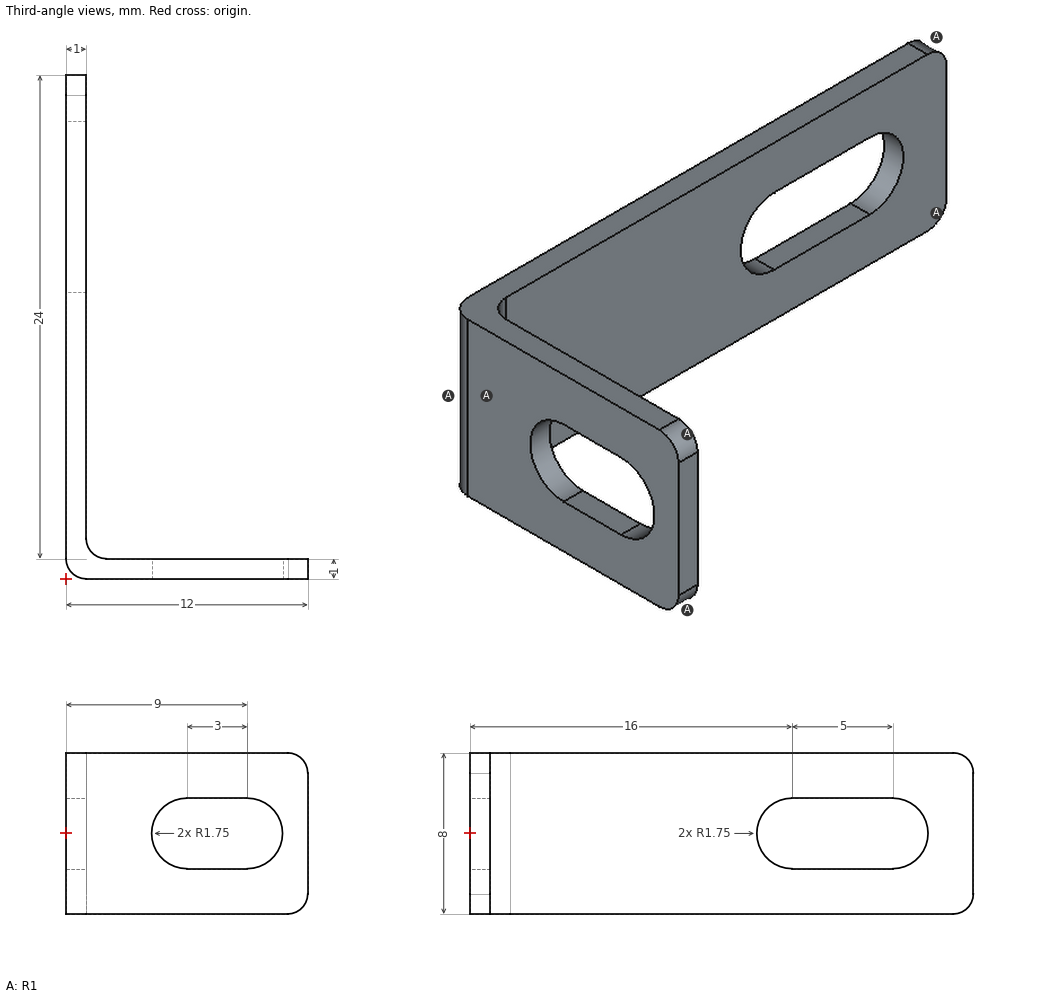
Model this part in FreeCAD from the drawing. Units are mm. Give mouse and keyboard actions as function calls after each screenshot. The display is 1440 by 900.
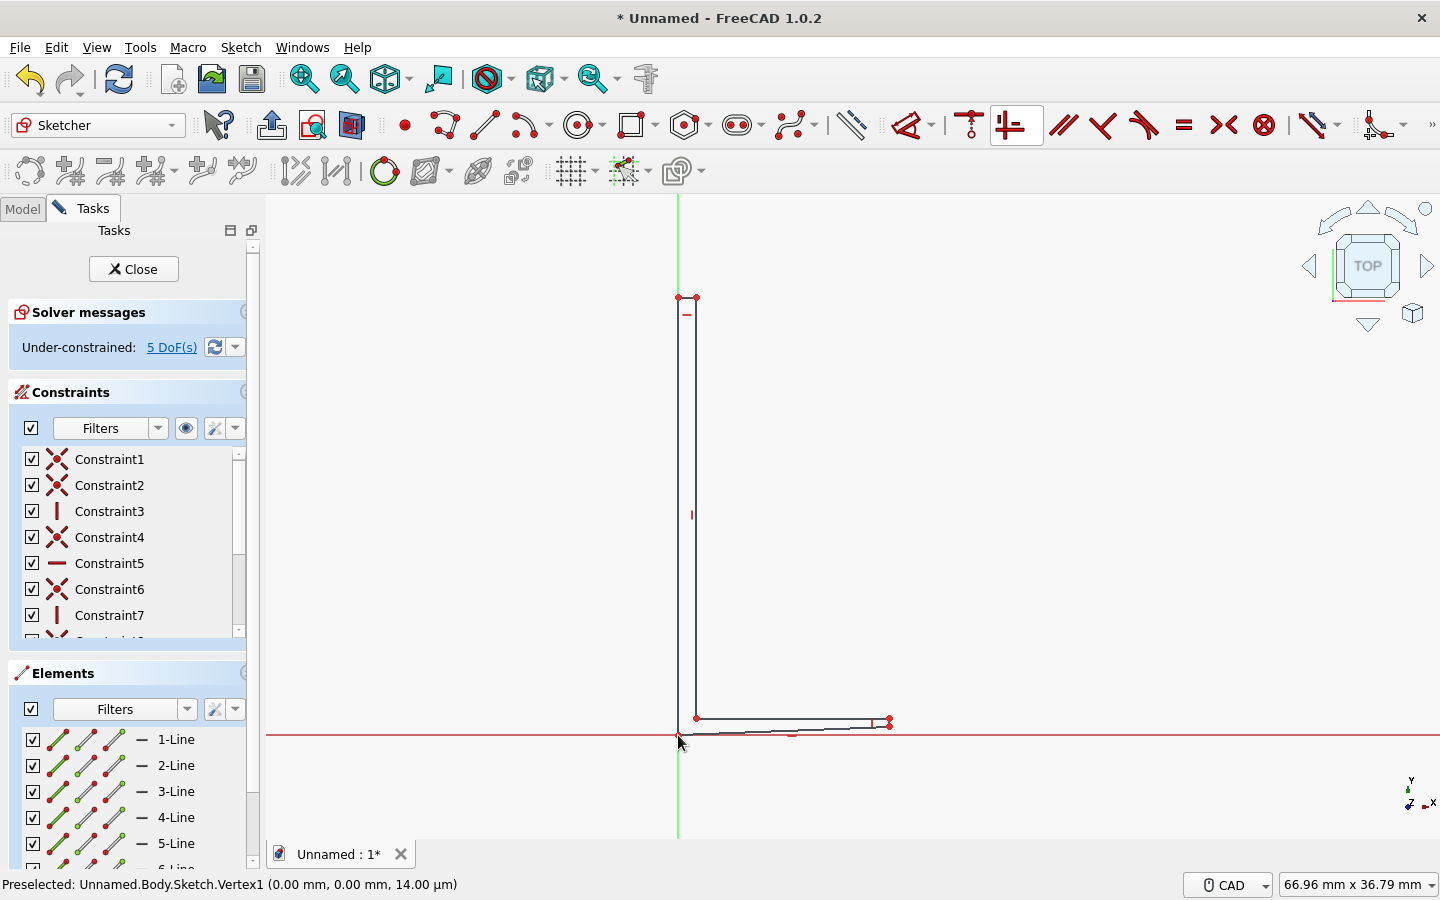
click(742, 733)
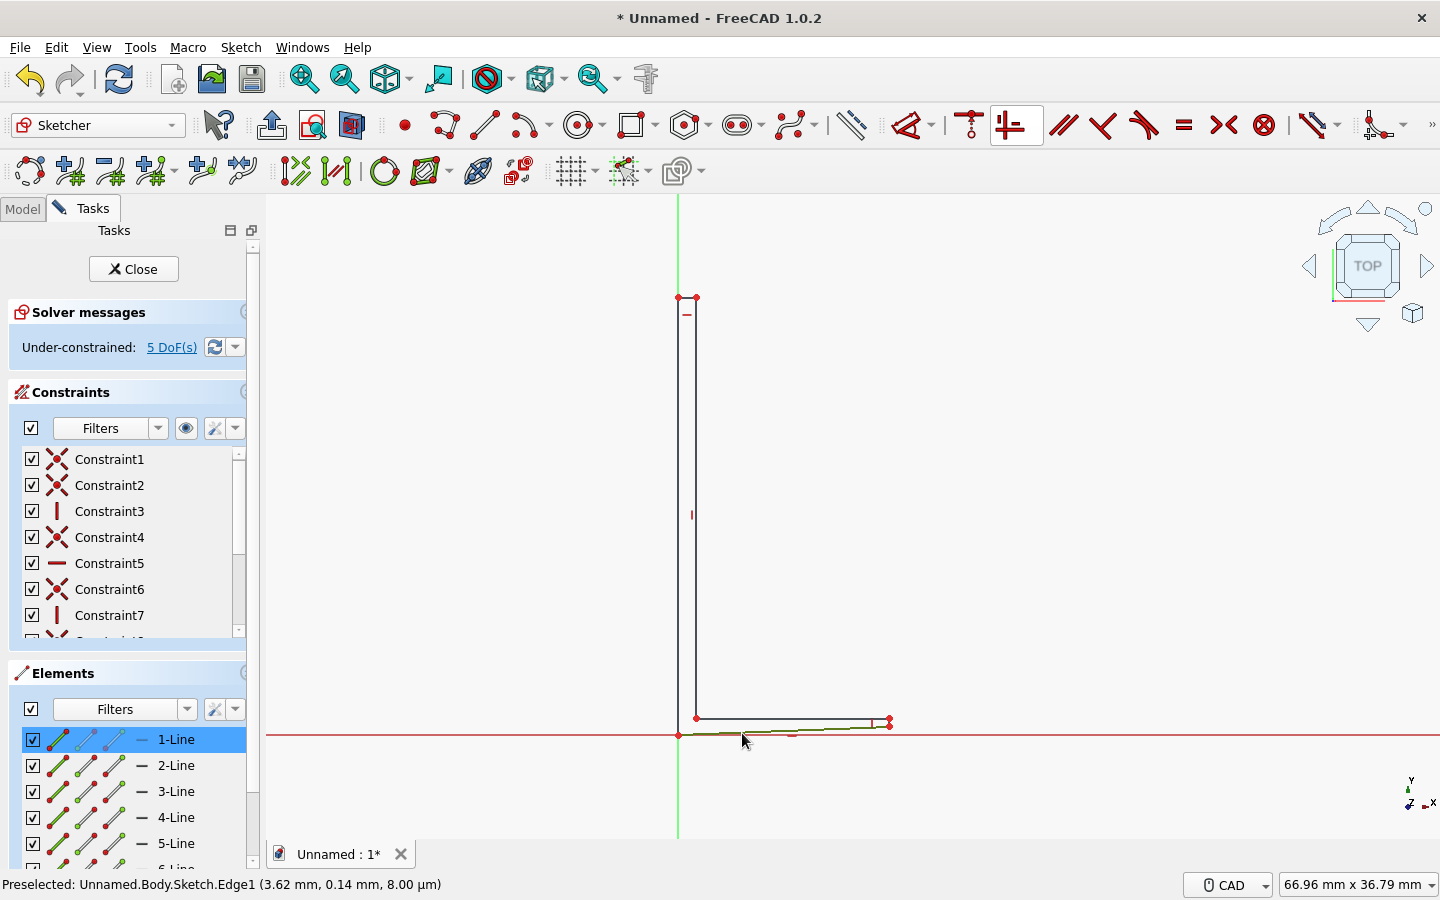
key(h)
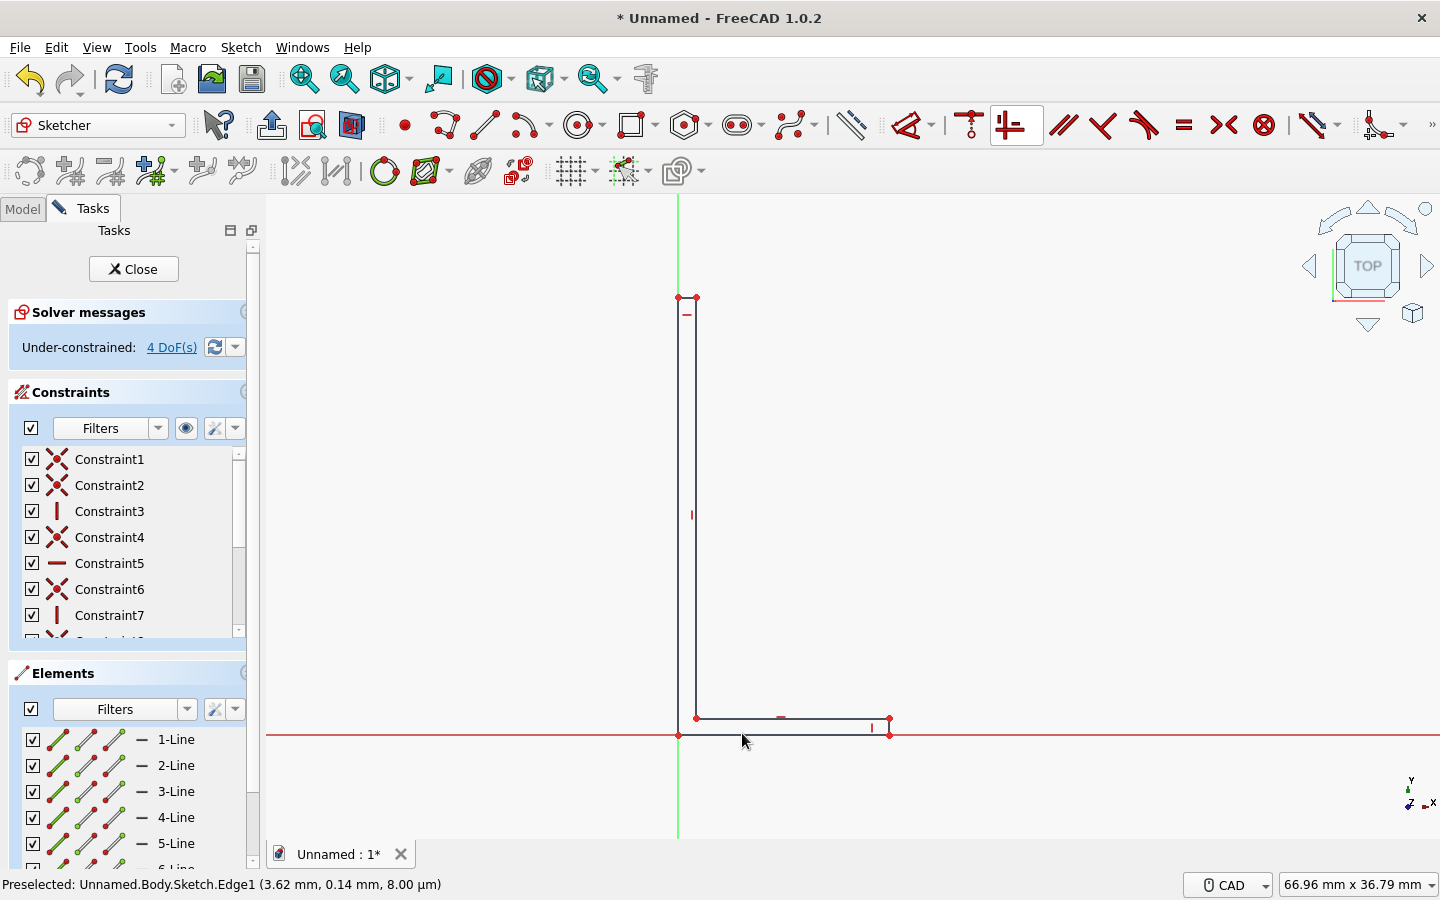
key(d)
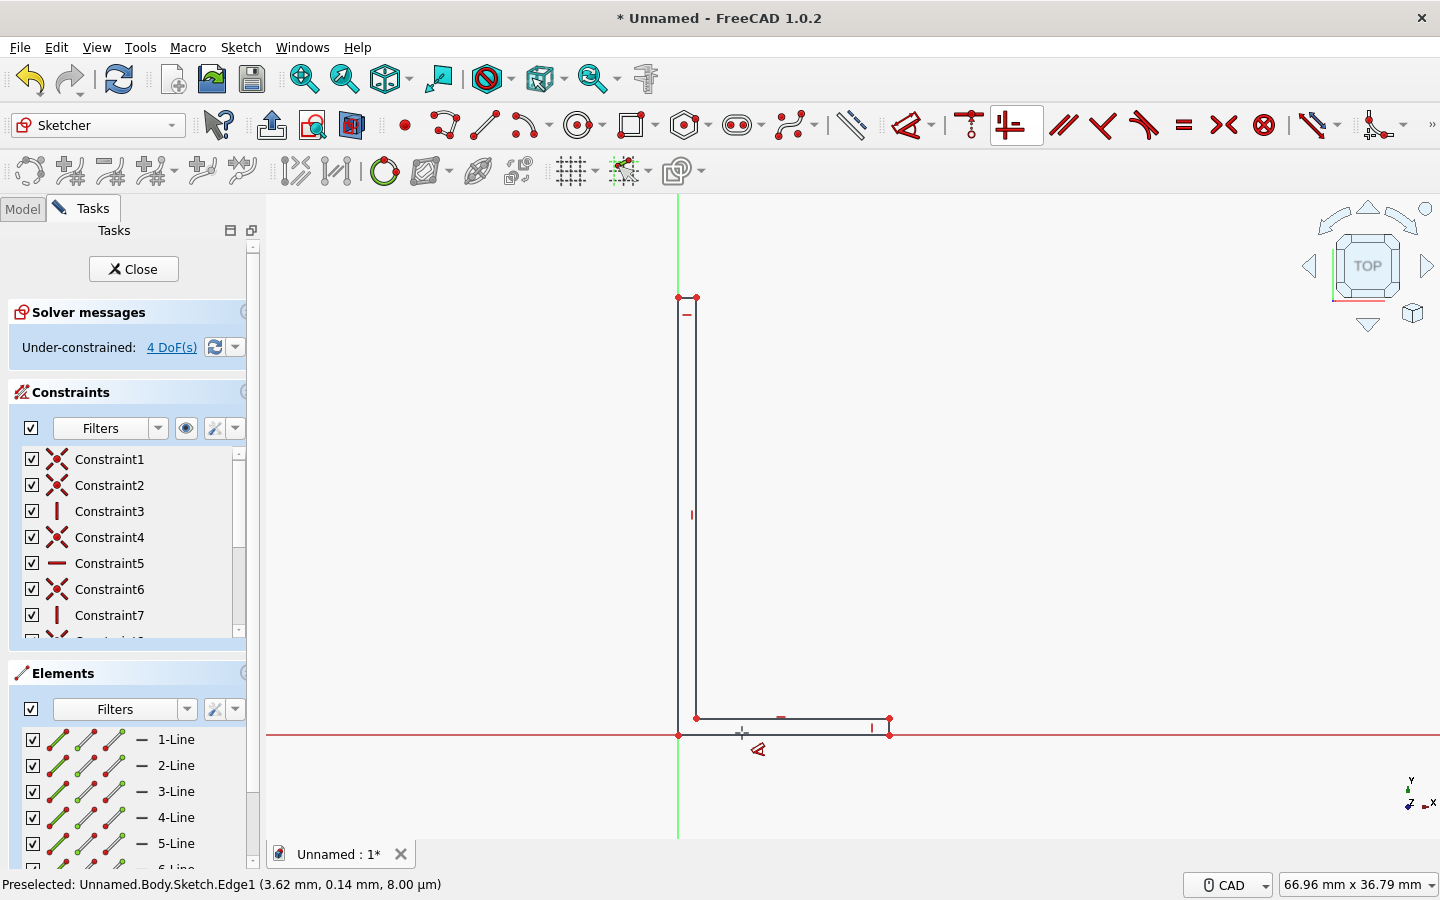
scroll(889, 727, up, 5)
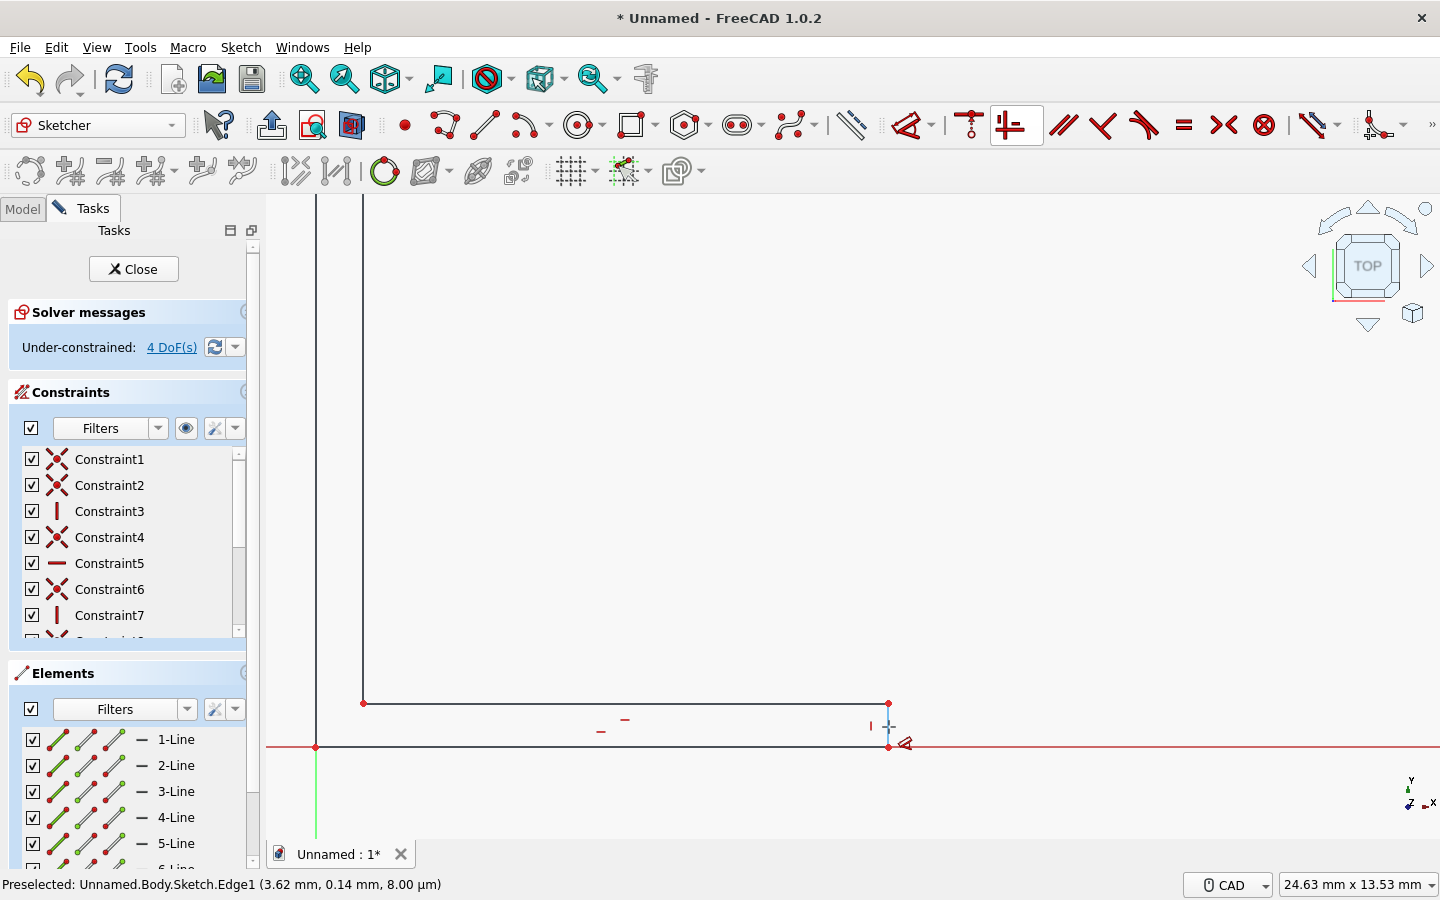
click(888, 726)
click(922, 726)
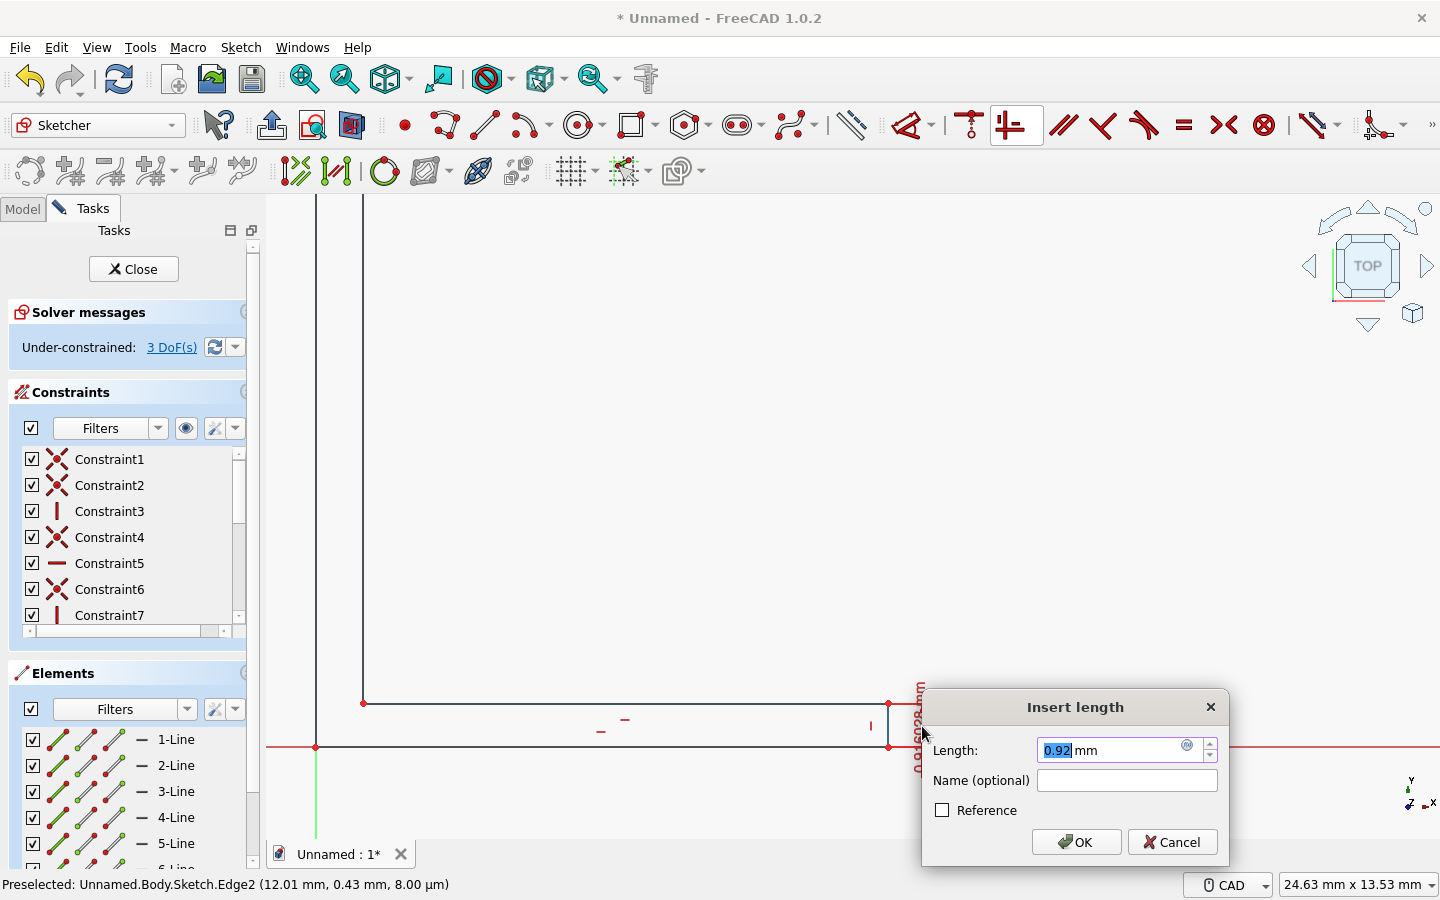
text(1)
key(Return)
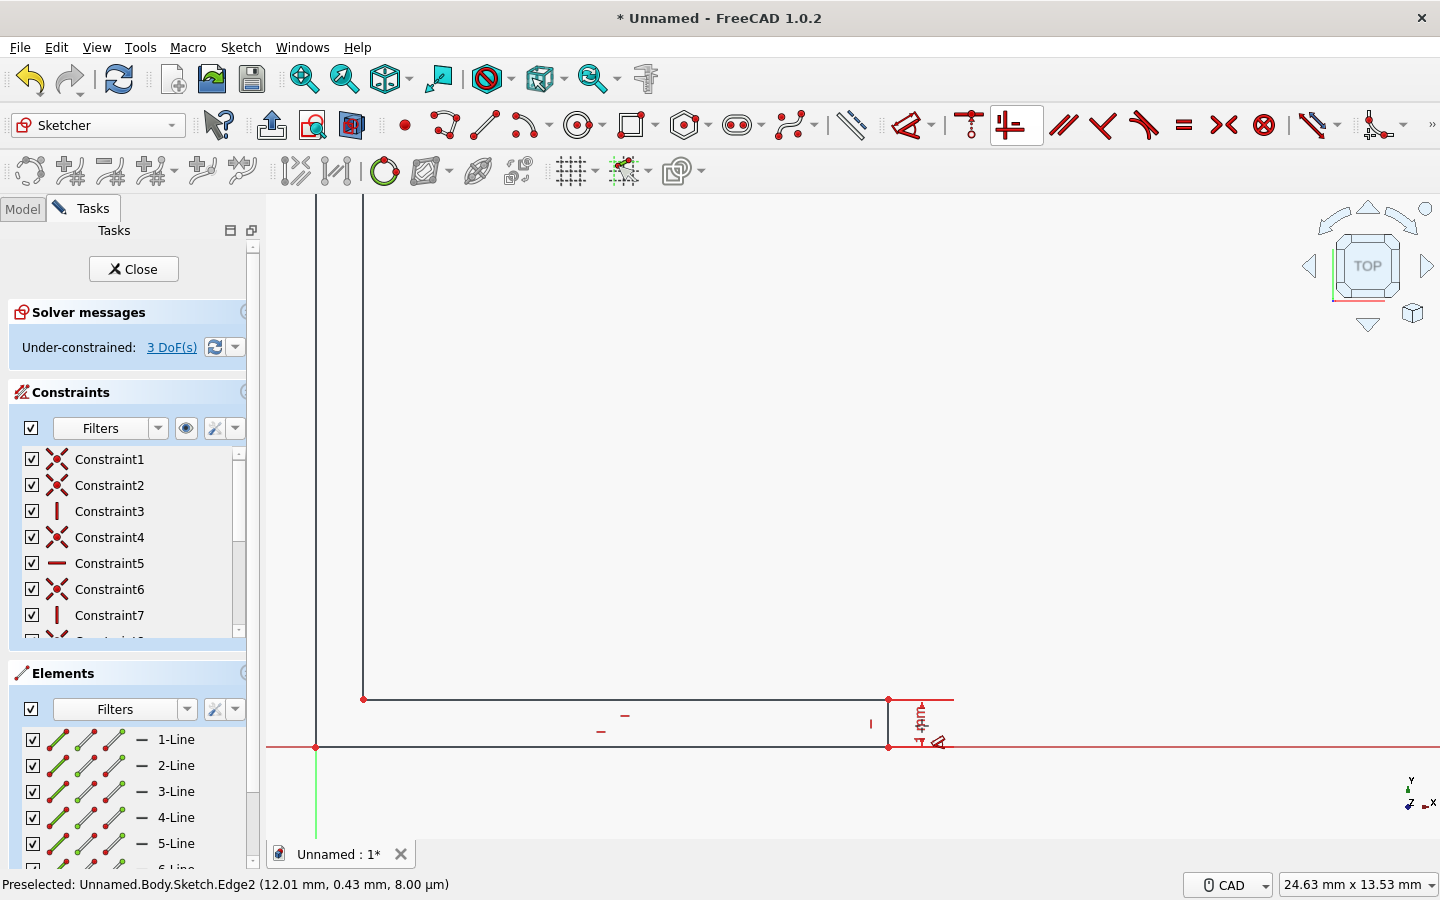
scroll(891, 729, down, 5)